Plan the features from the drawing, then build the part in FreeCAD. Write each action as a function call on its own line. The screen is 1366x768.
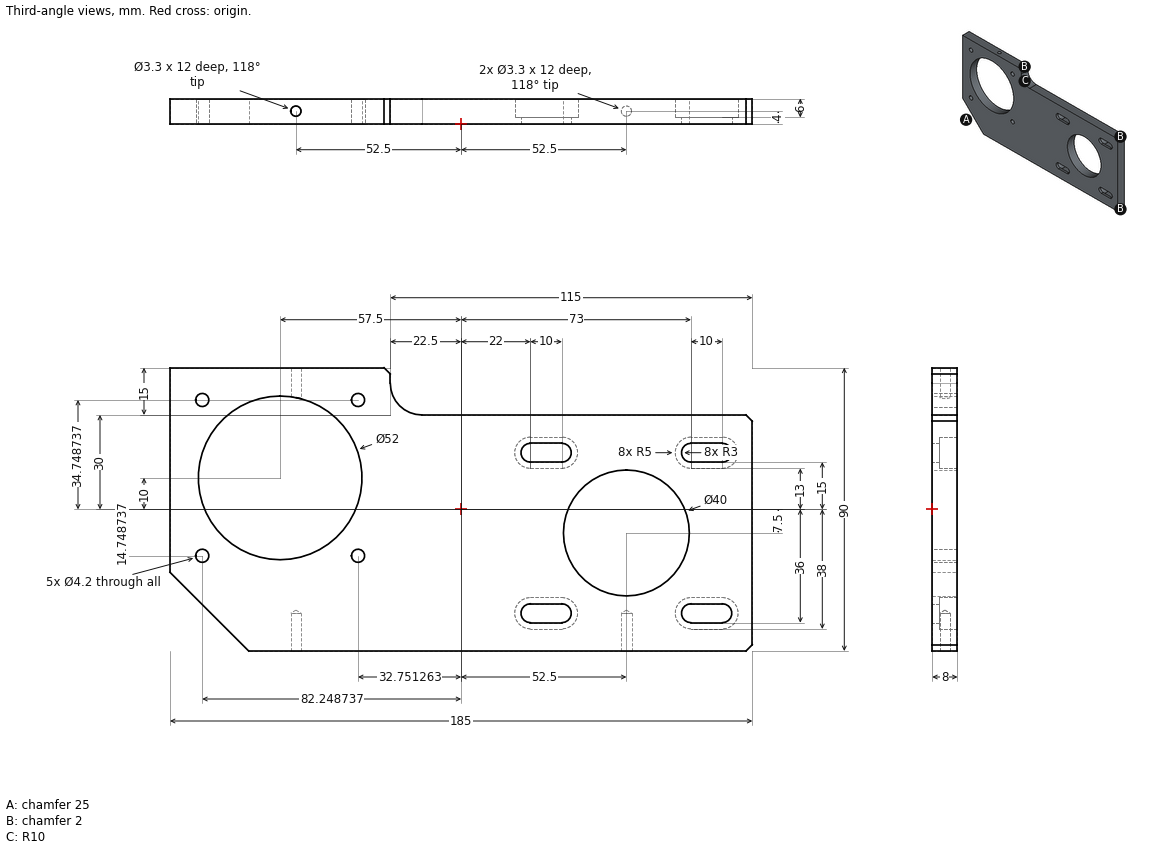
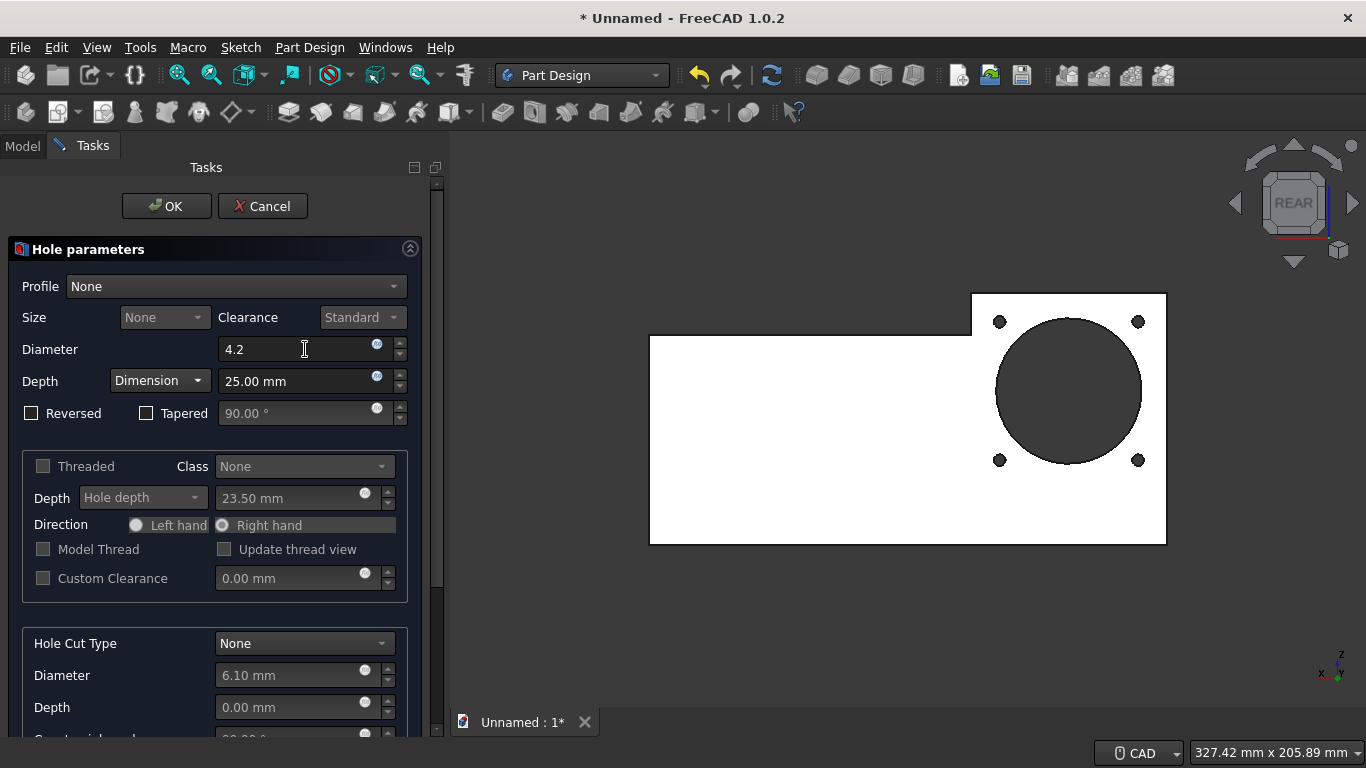
click(161, 380)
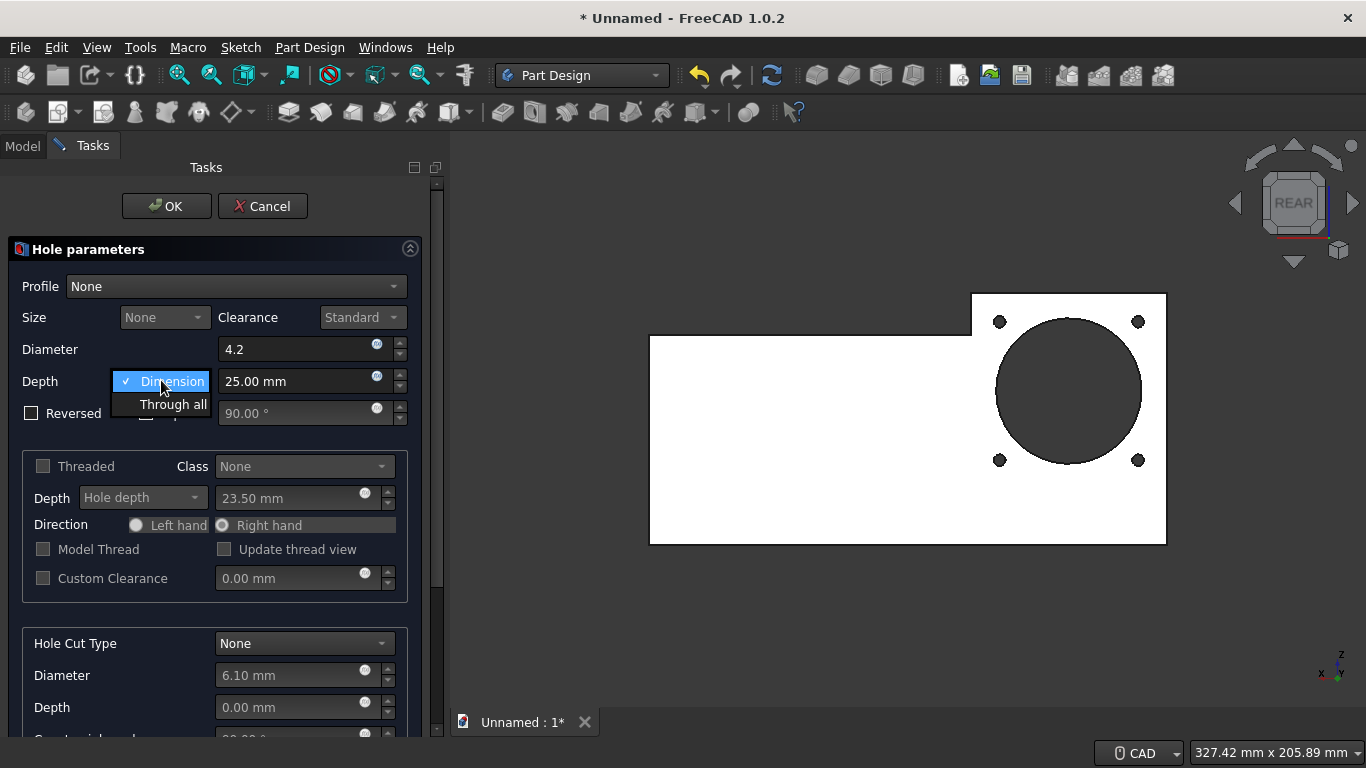
click(160, 404)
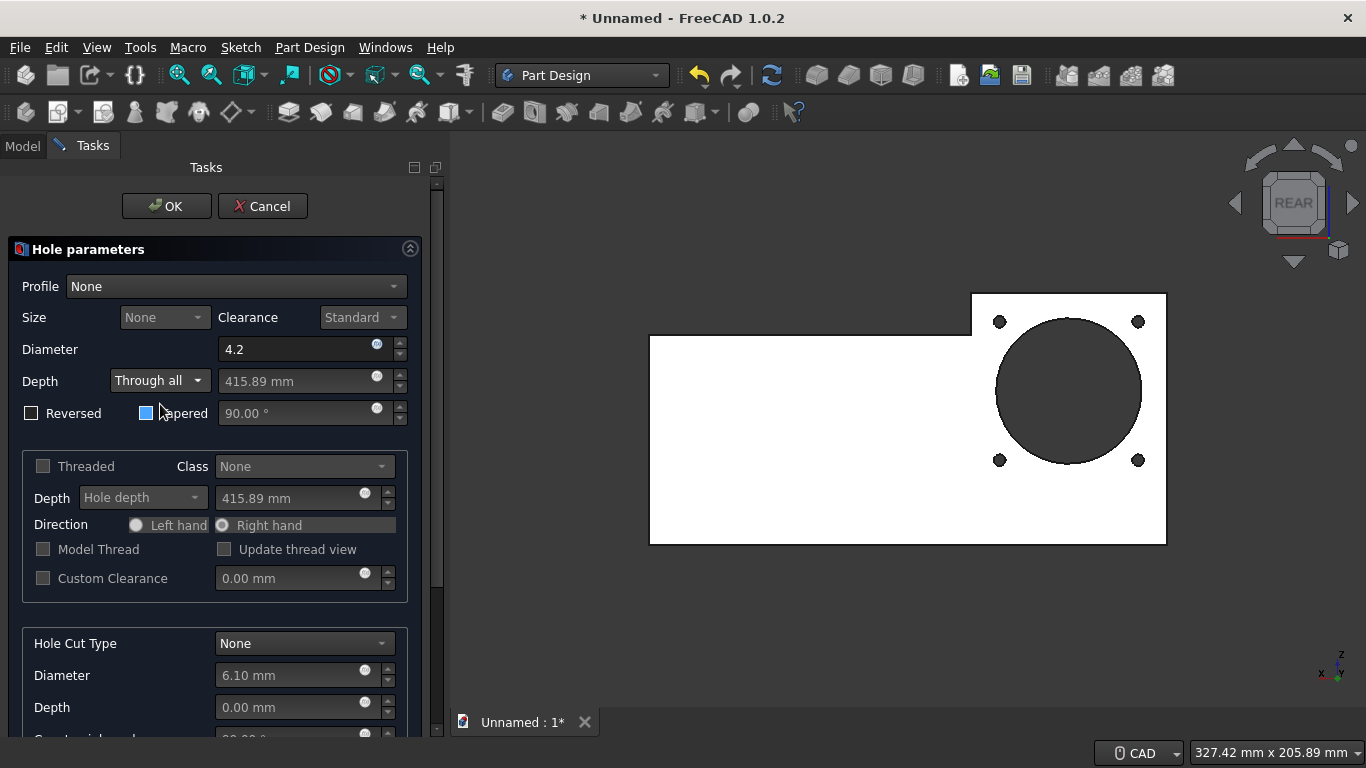
click(167, 206)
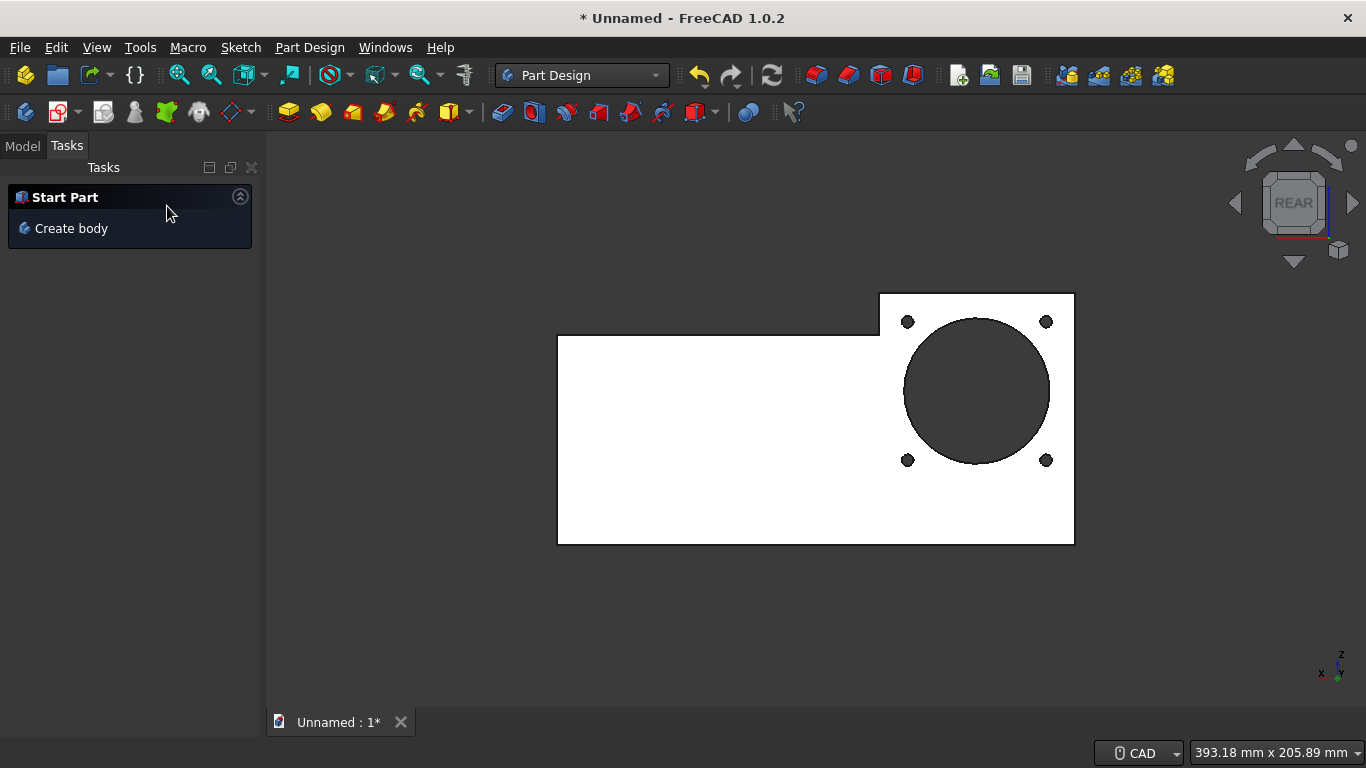
click(668, 454)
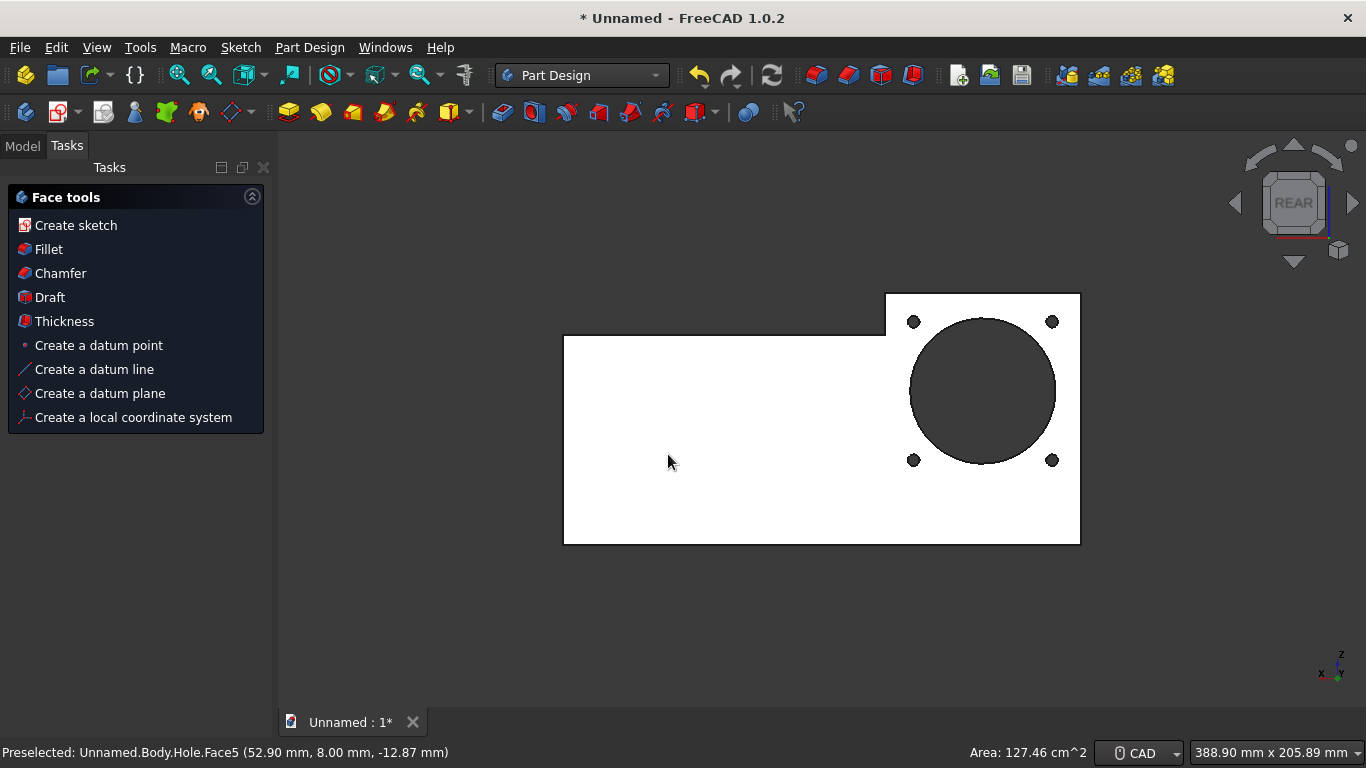
click(58, 112)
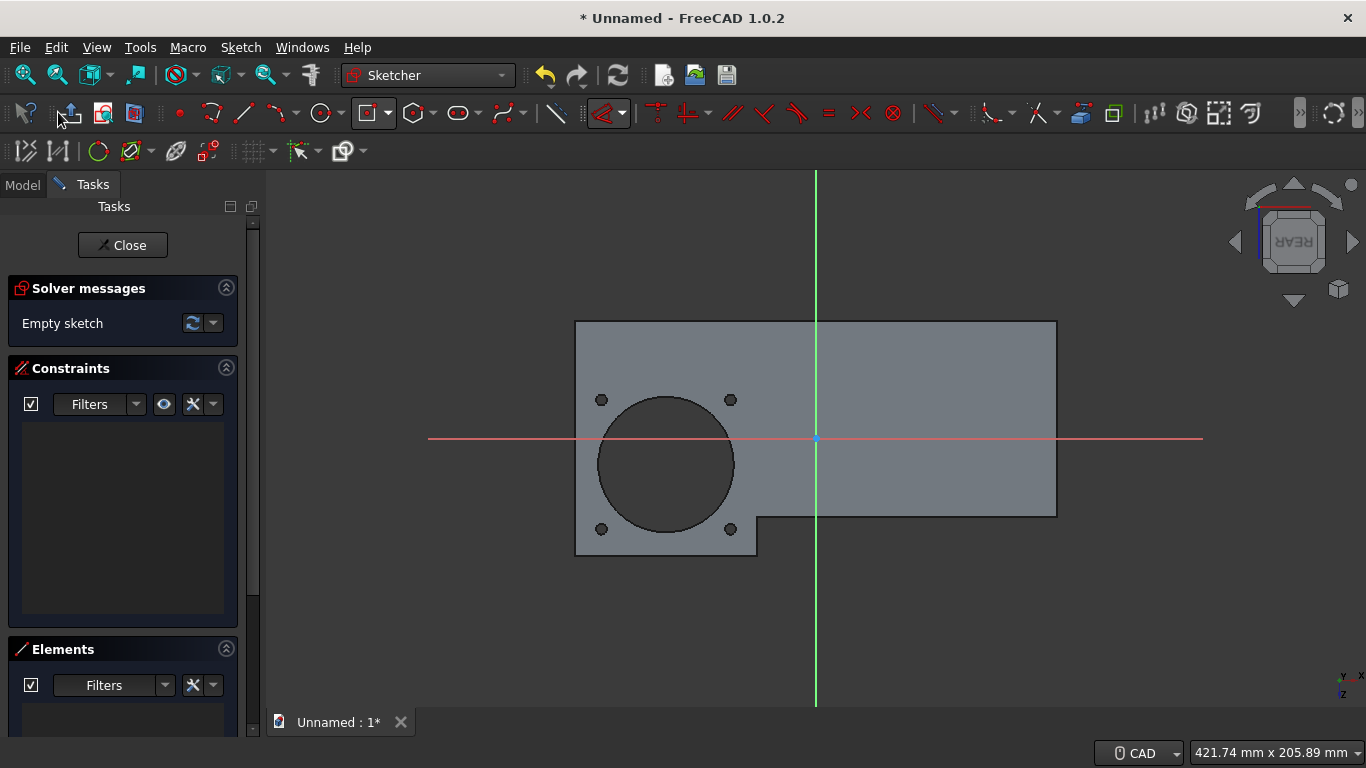
scroll(981, 411, up, 6)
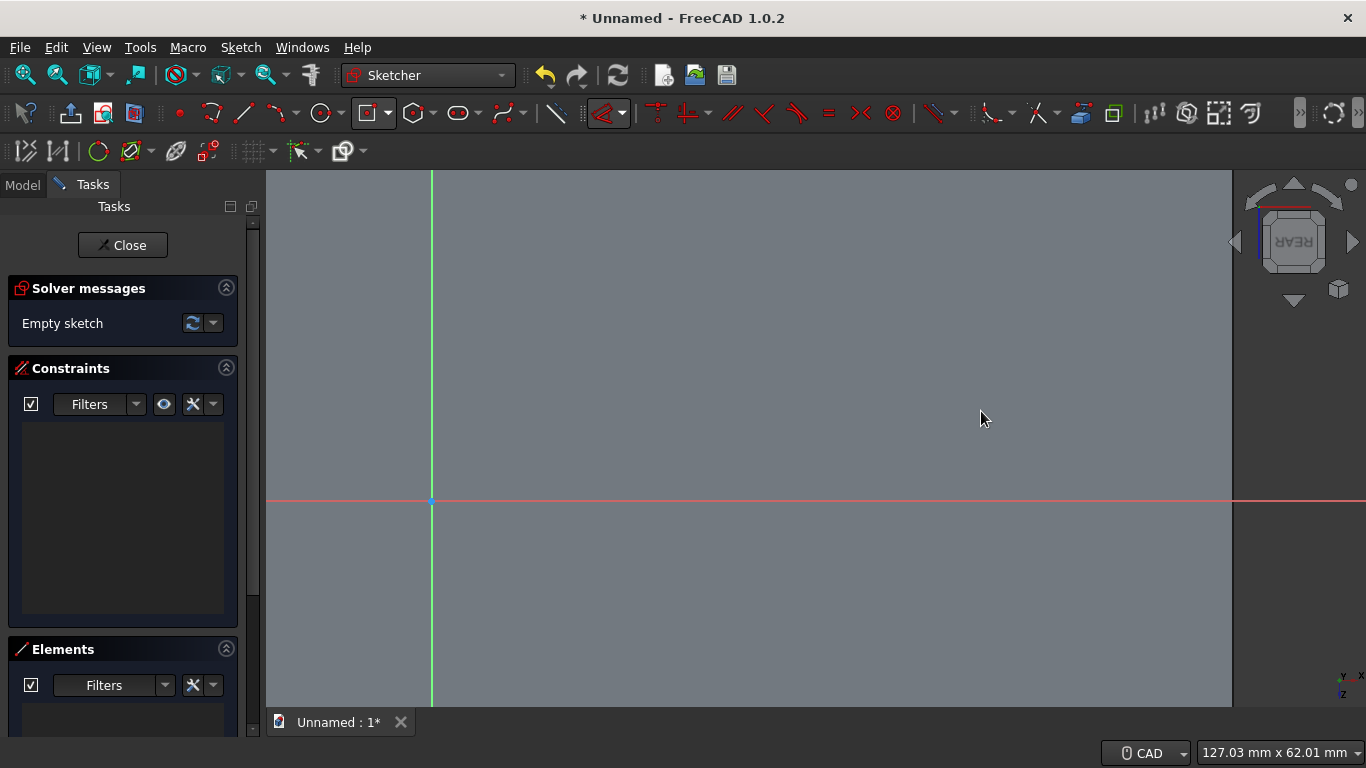
key(g)
key(c)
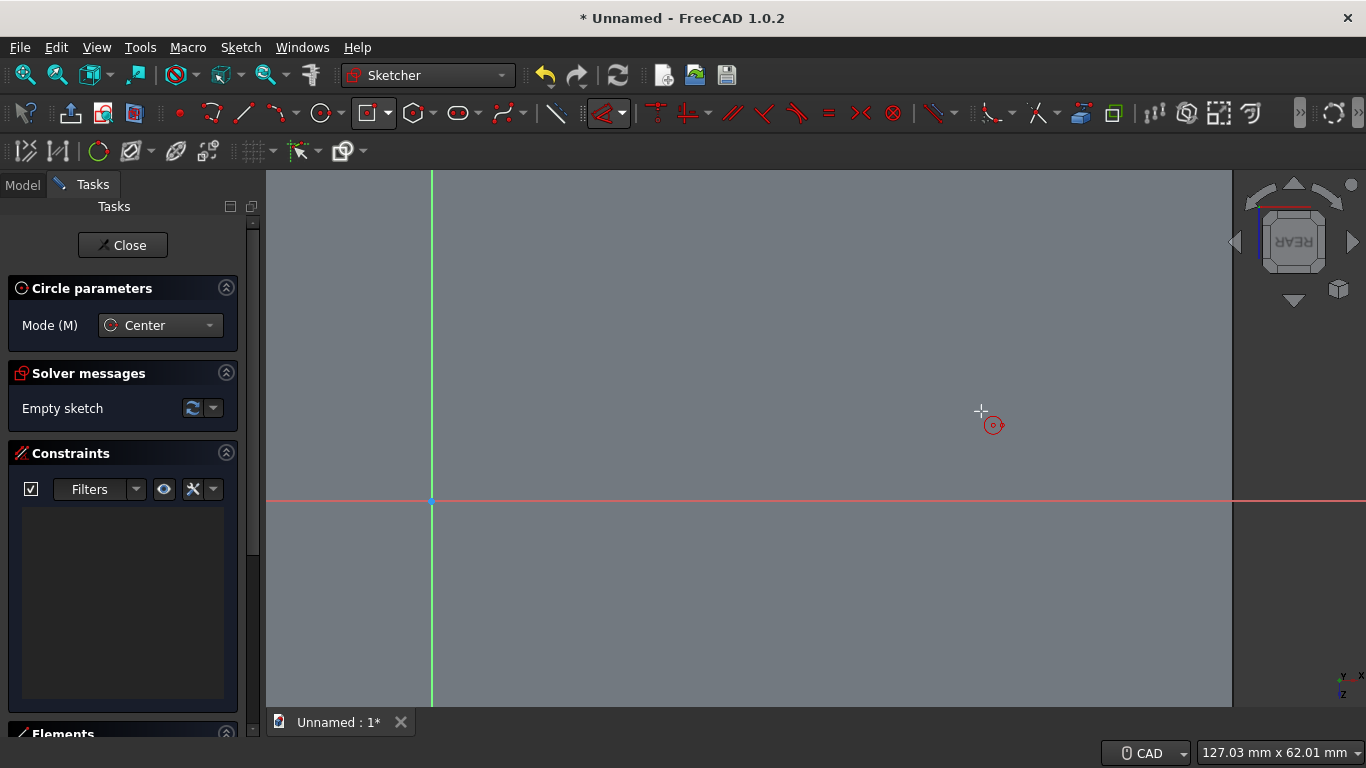
click(886, 436)
click(1009, 314)
key(Escape)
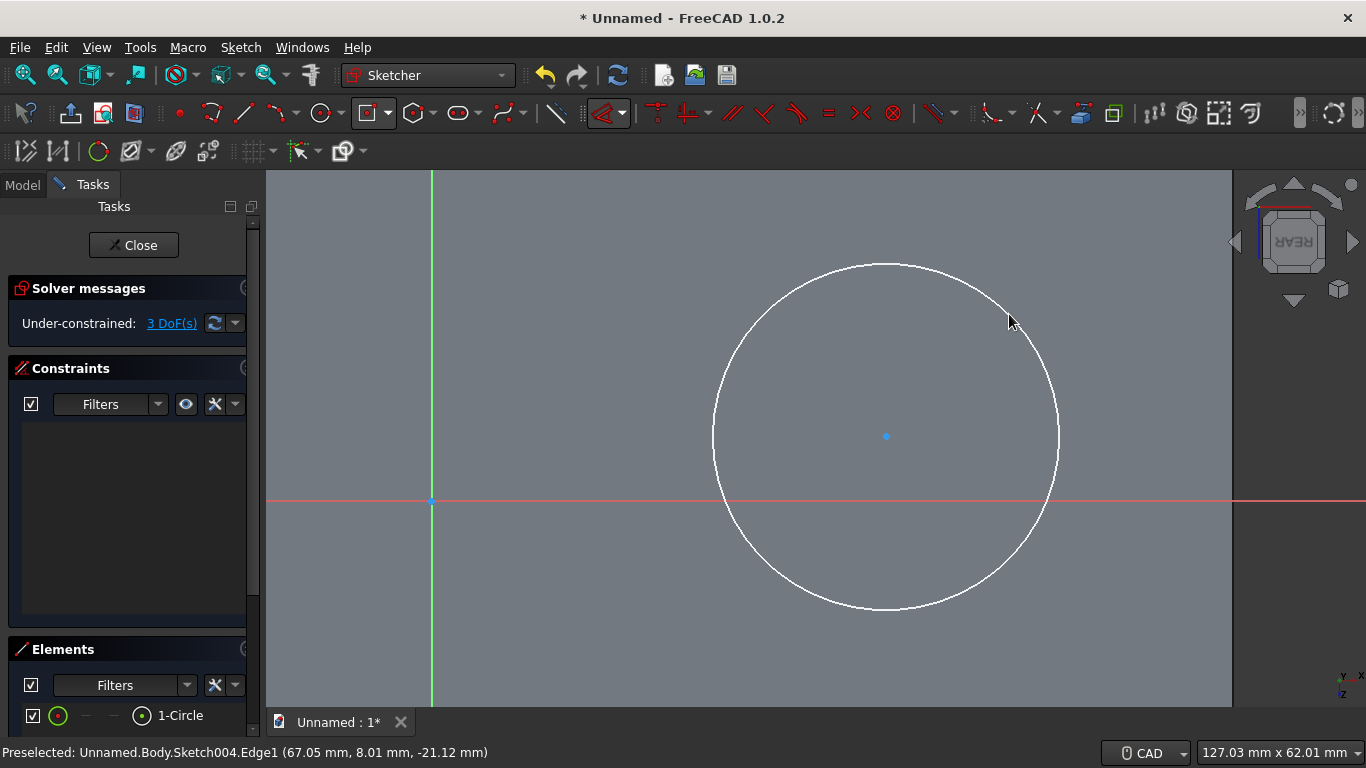
click(1008, 314)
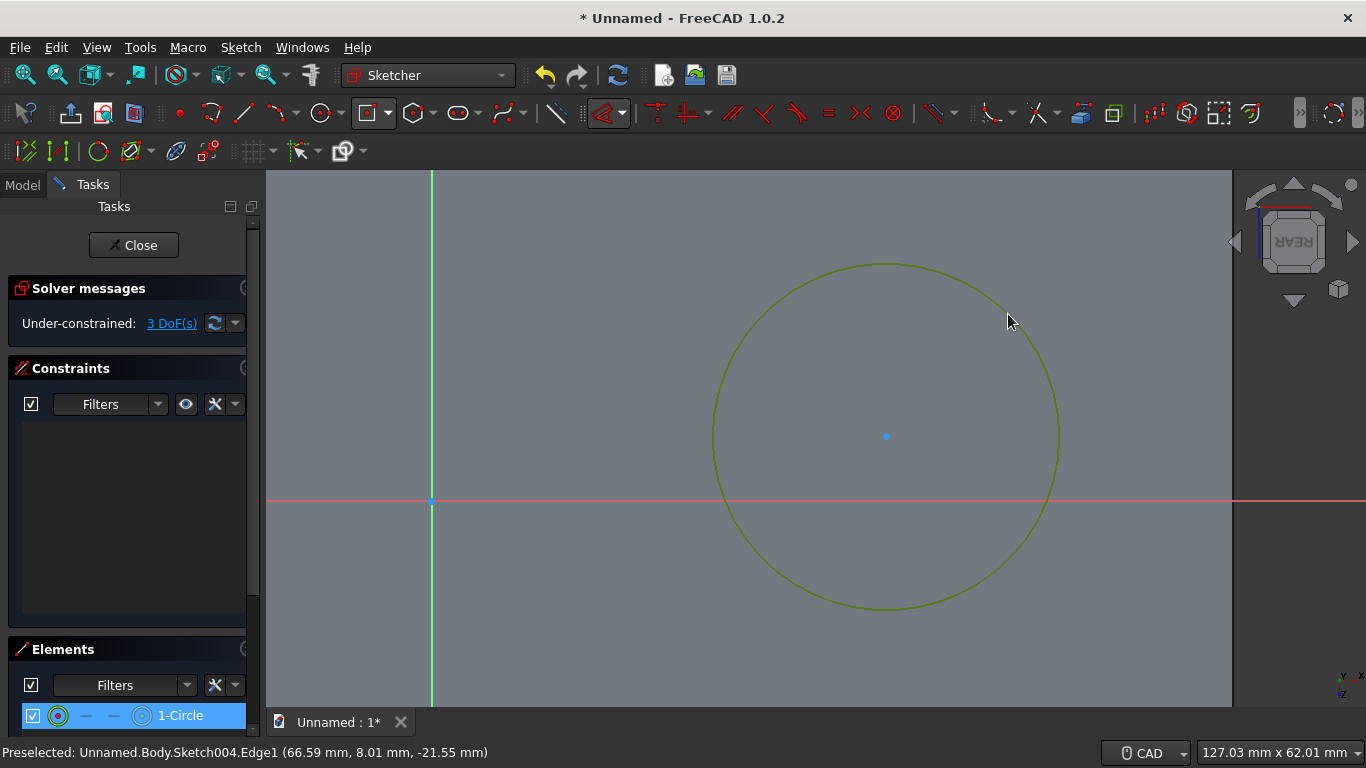
key(k)
key(o)